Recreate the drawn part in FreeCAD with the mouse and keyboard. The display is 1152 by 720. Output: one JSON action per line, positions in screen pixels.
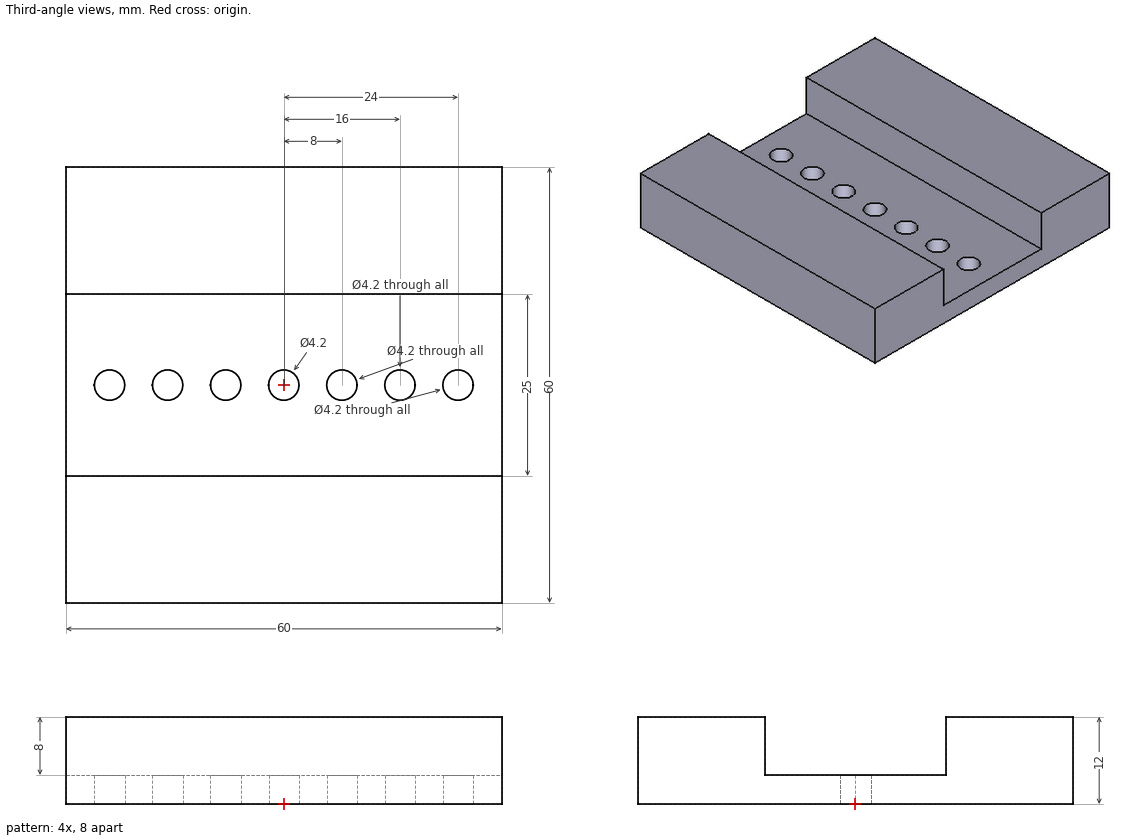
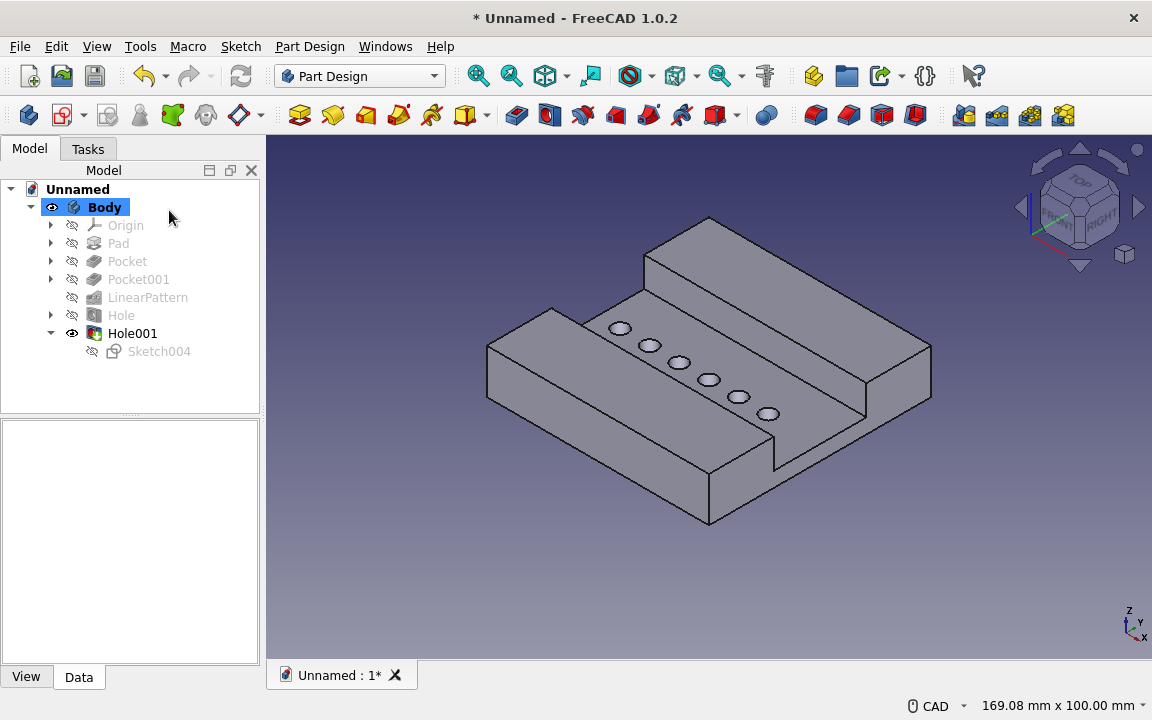
{"action": "left_click", "coordinate": [799, 400]}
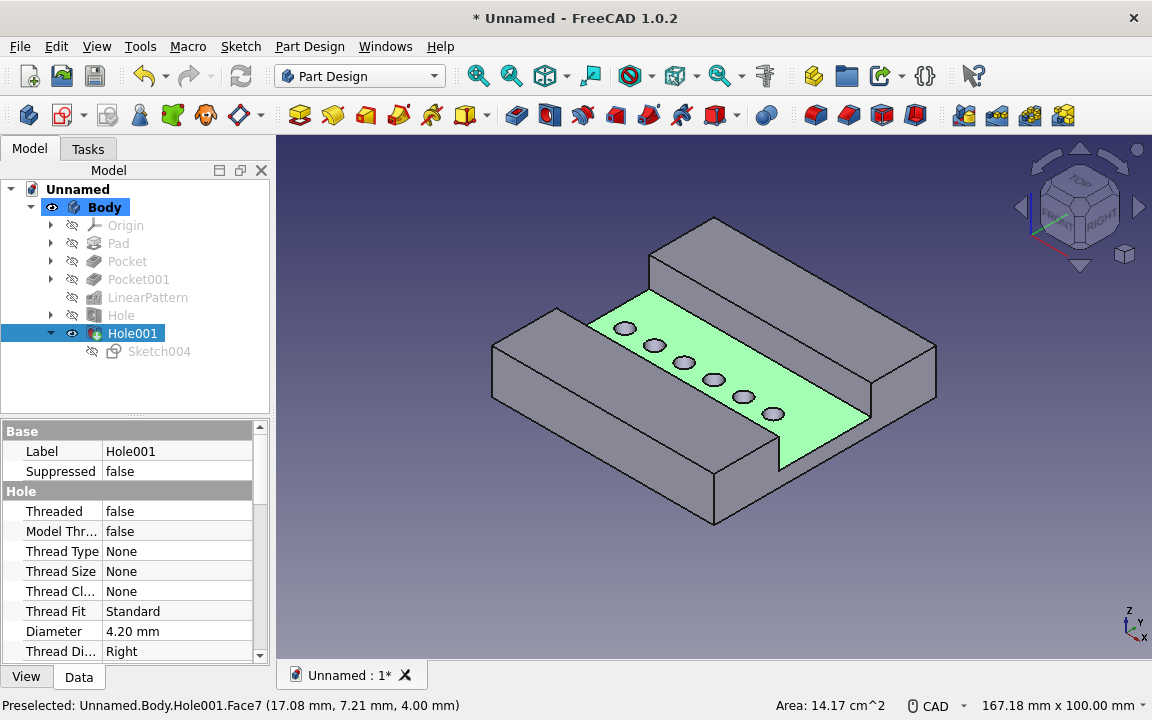
{"action": "left_click", "coordinate": [62, 116]}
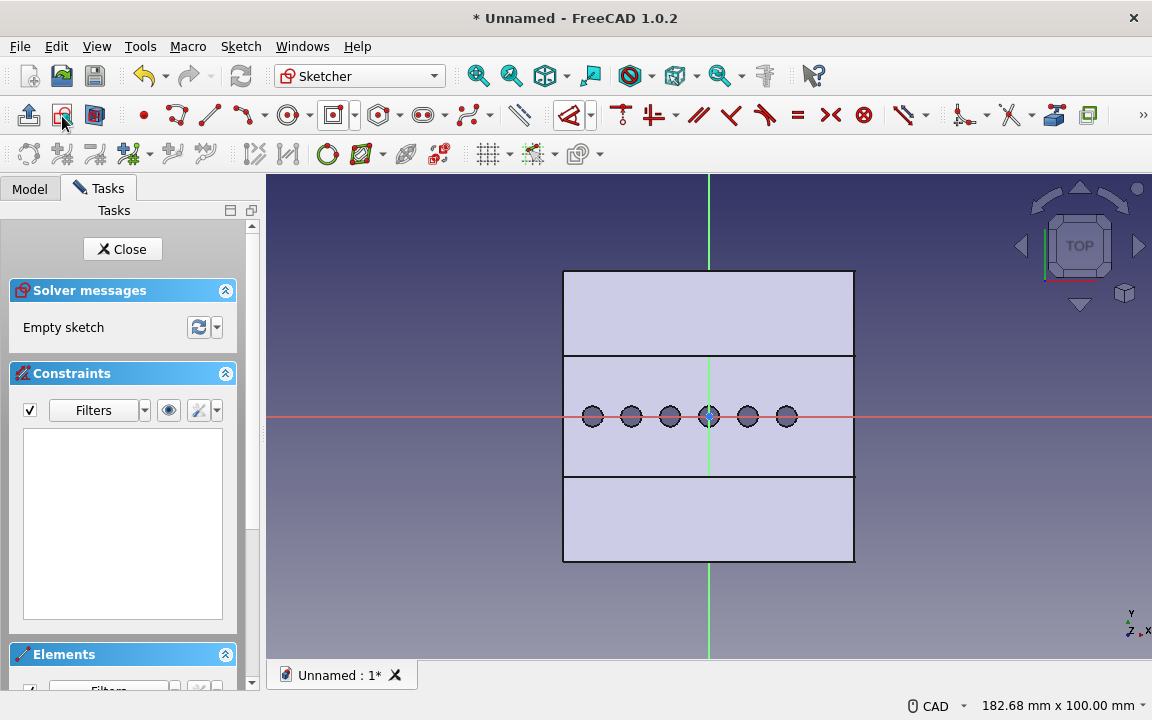
{"action": "left_click", "coordinate": [95, 116]}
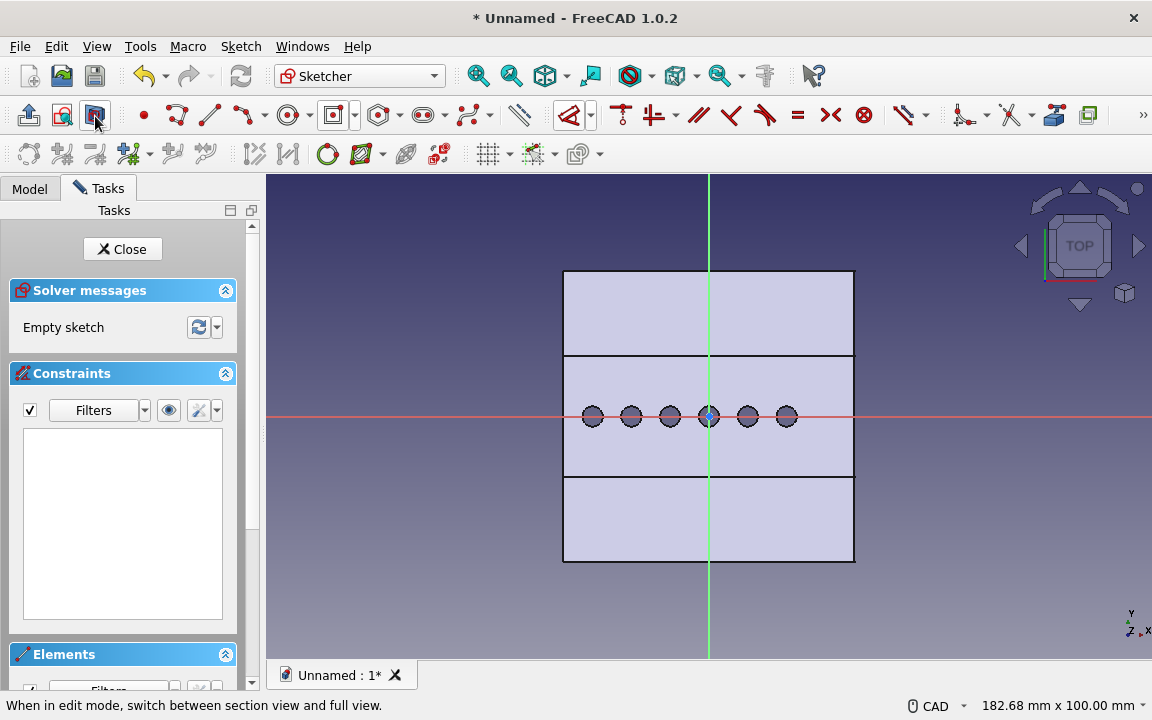
{"action": "scroll", "coordinate": [840, 416], "scroll_direction": "up", "scroll_amount": 13}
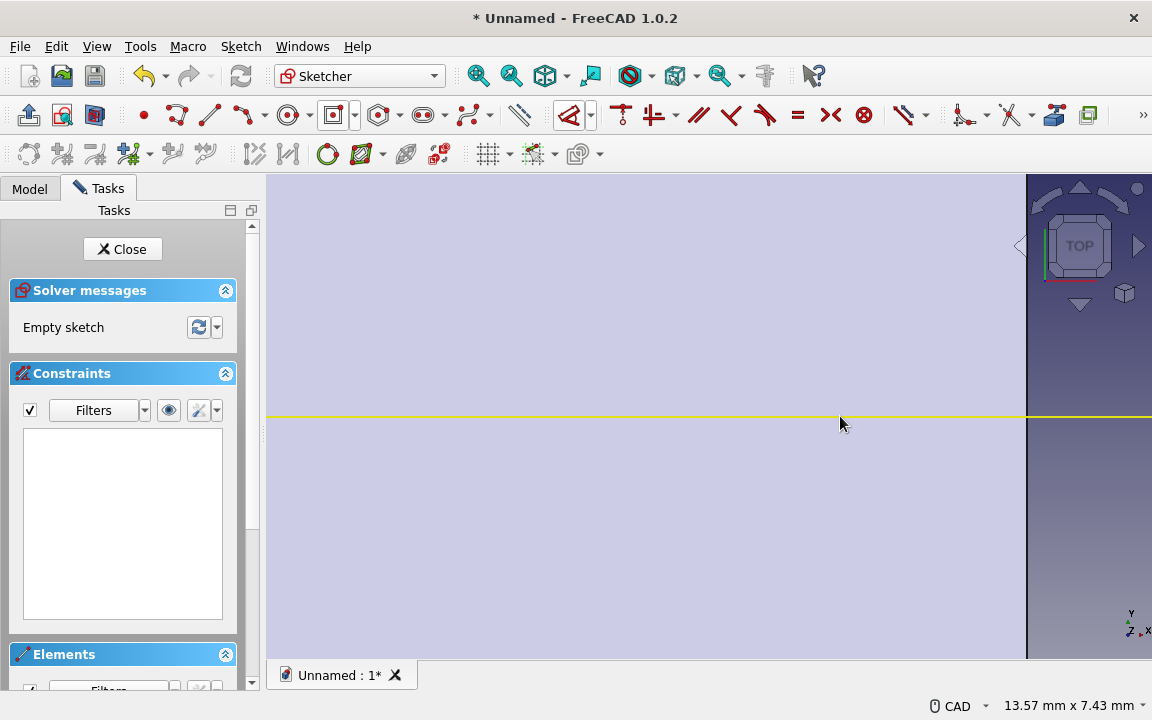
{"action": "left_click", "coordinate": [288, 116]}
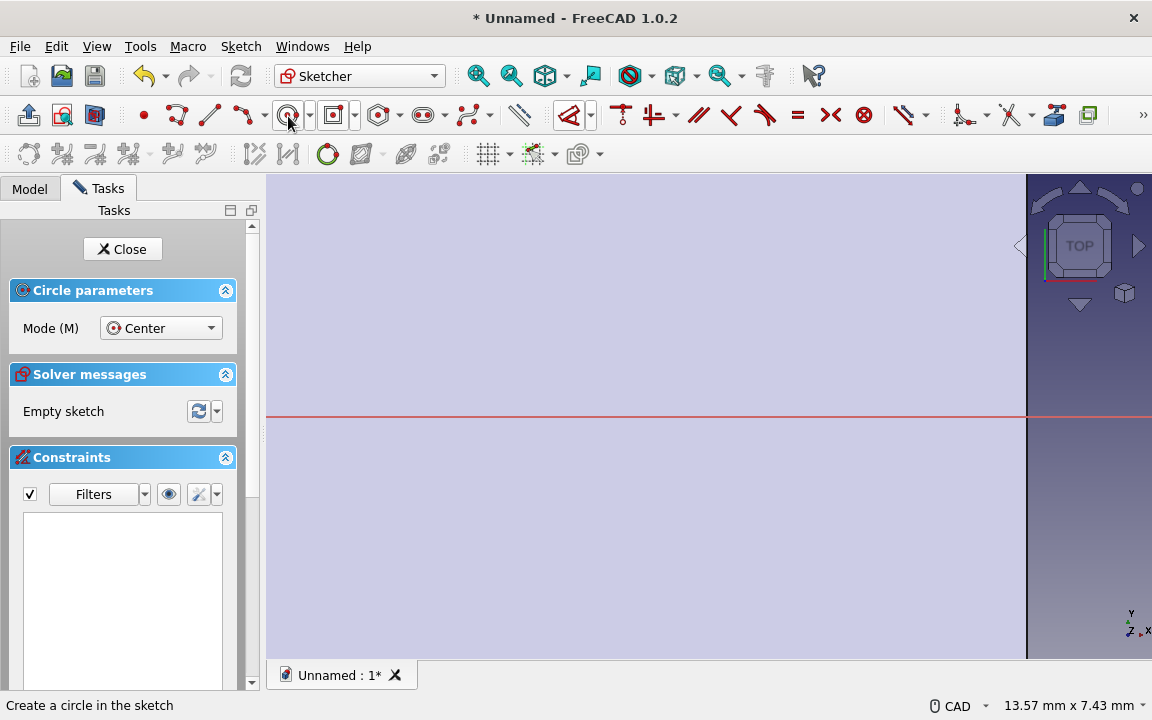
{"action": "left_click", "coordinate": [635, 416]}
{"action": "mouse_move", "coordinate": [732, 320]}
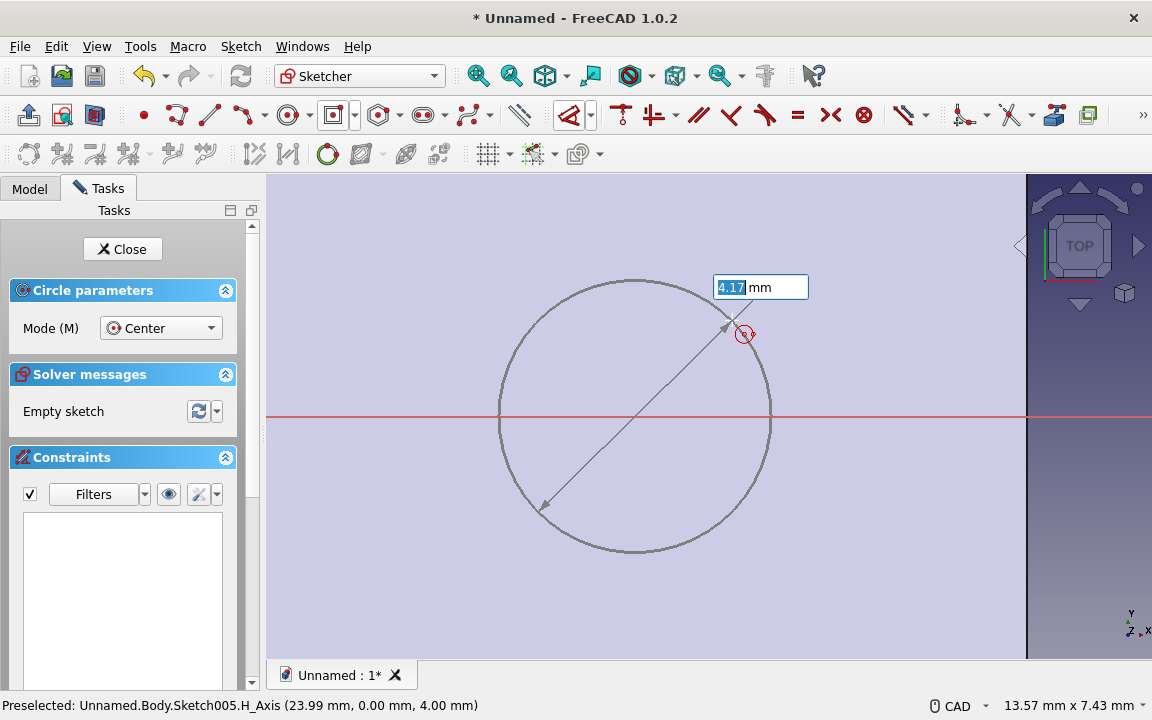
{"action": "type", "text": "4.2"}
{"action": "key", "text": "Return"}
{"action": "key", "text": "Escape"}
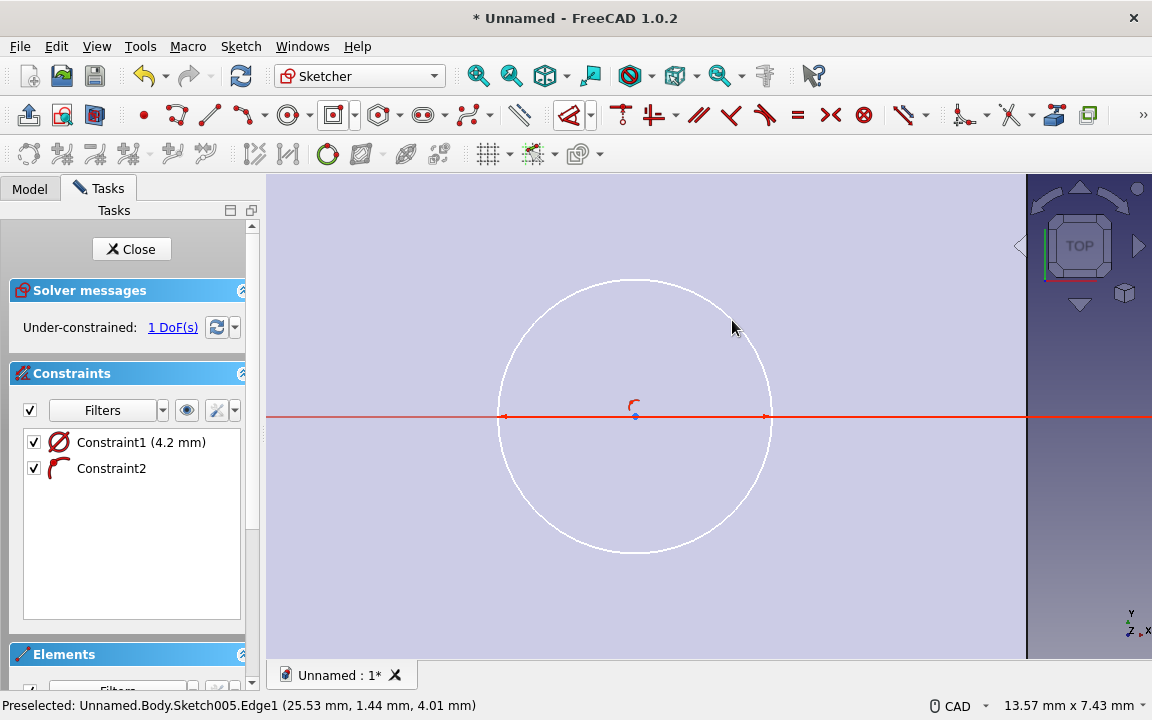
{"action": "left_click", "coordinate": [635, 416]}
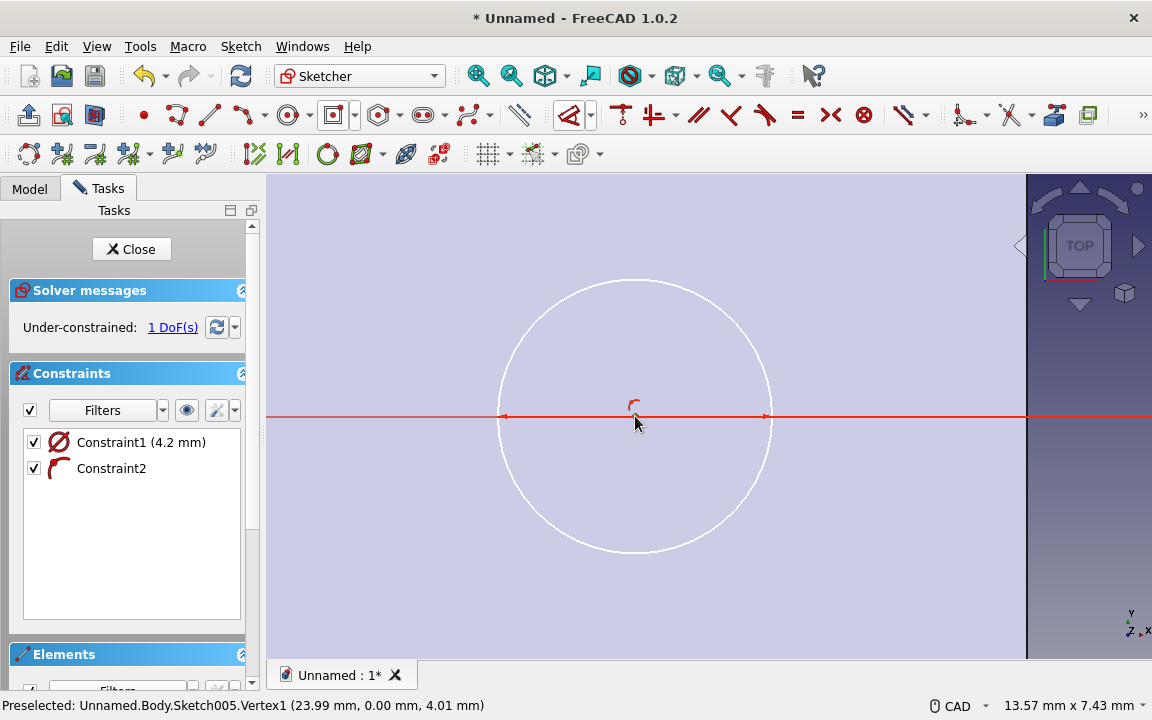
{"action": "left_click", "coordinate": [590, 116]}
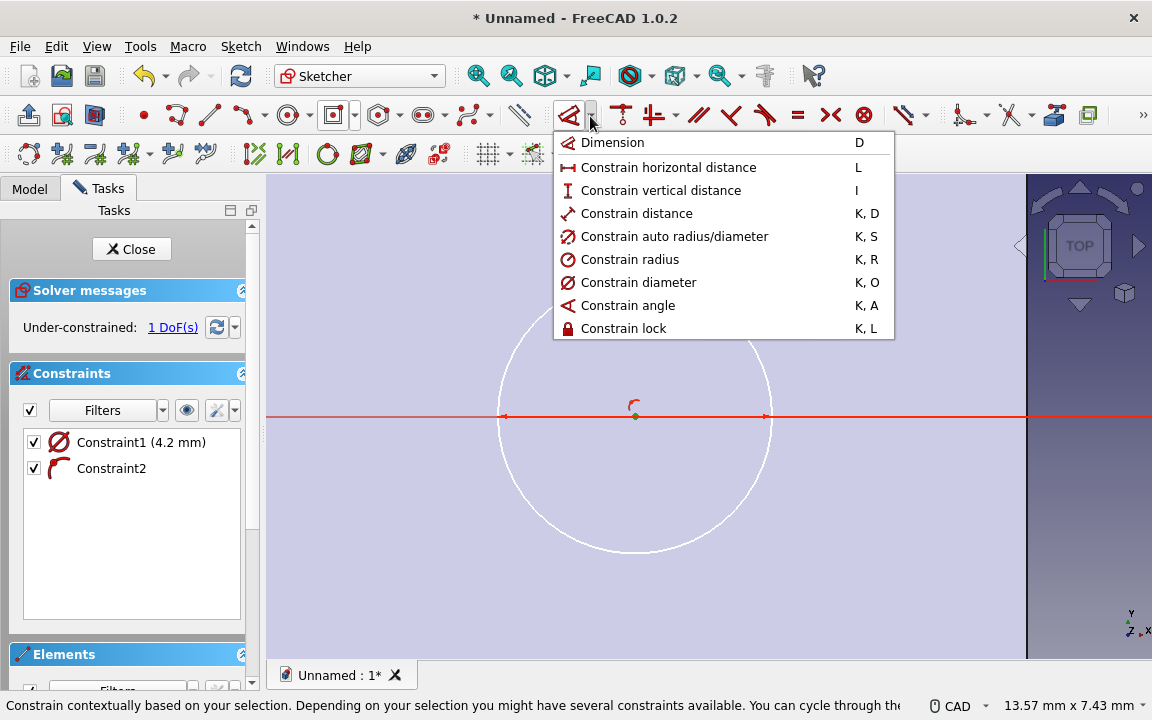
{"action": "left_click", "coordinate": [724, 168]}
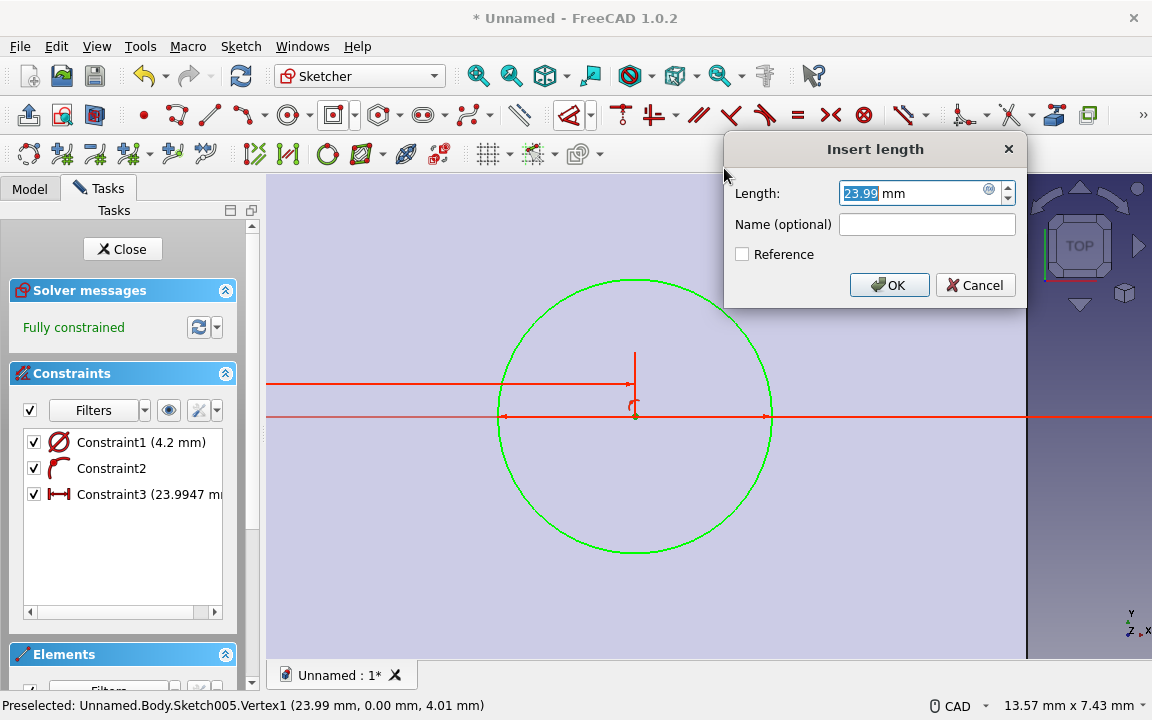
{"action": "type", "text": "24"}
{"action": "key", "text": "Return"}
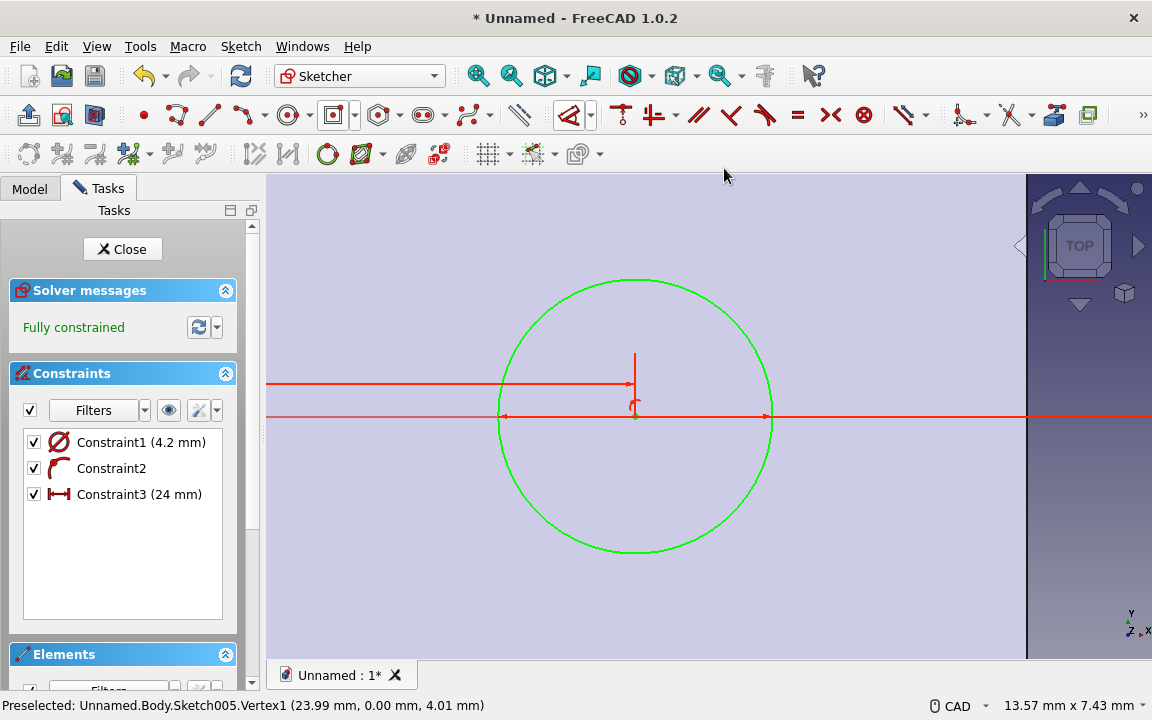
{"action": "left_click", "coordinate": [123, 249]}